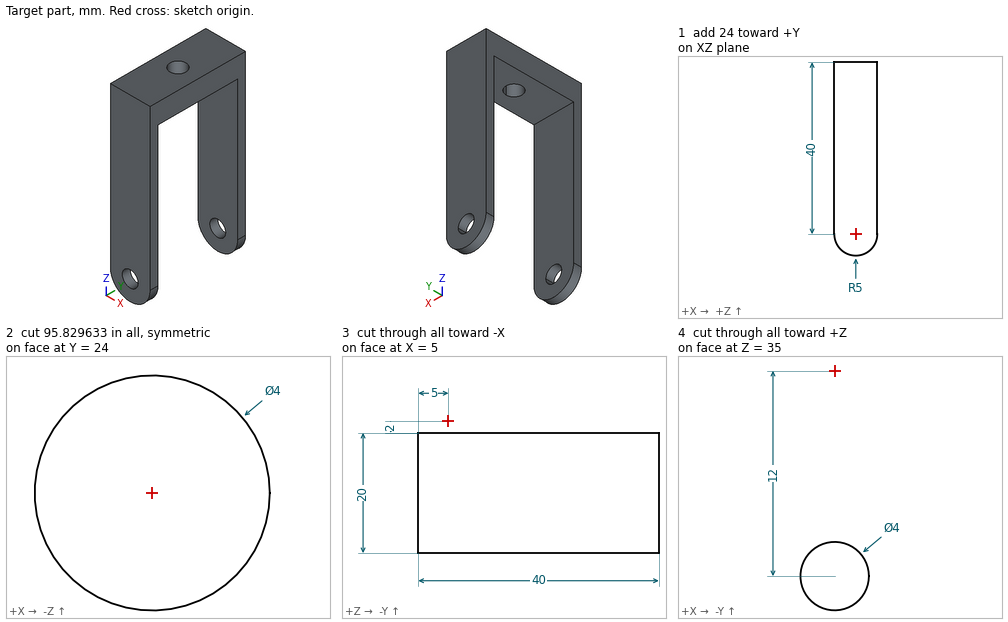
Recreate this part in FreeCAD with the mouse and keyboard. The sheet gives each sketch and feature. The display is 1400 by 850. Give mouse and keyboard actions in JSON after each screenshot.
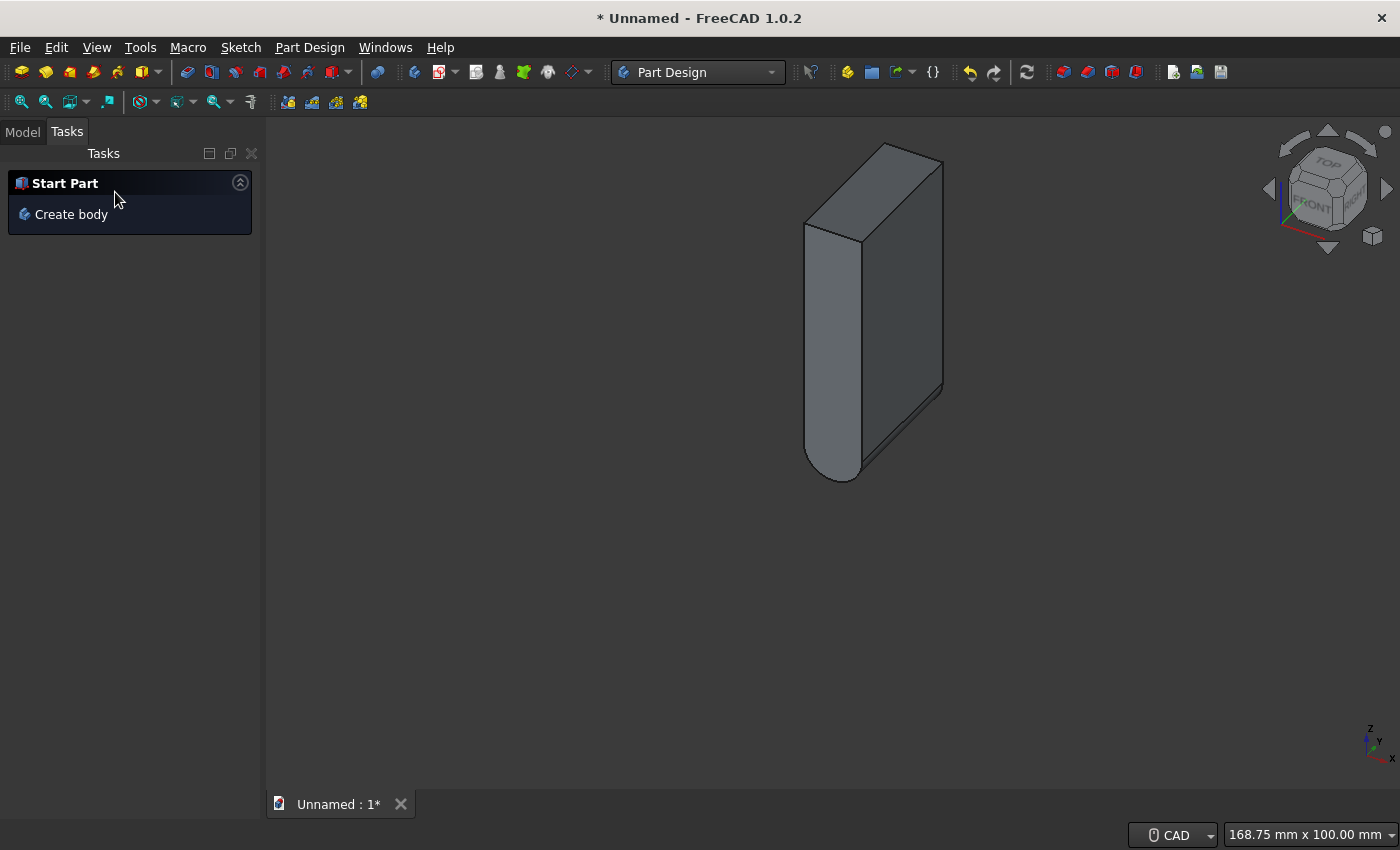
{"action": "key", "text": "4"}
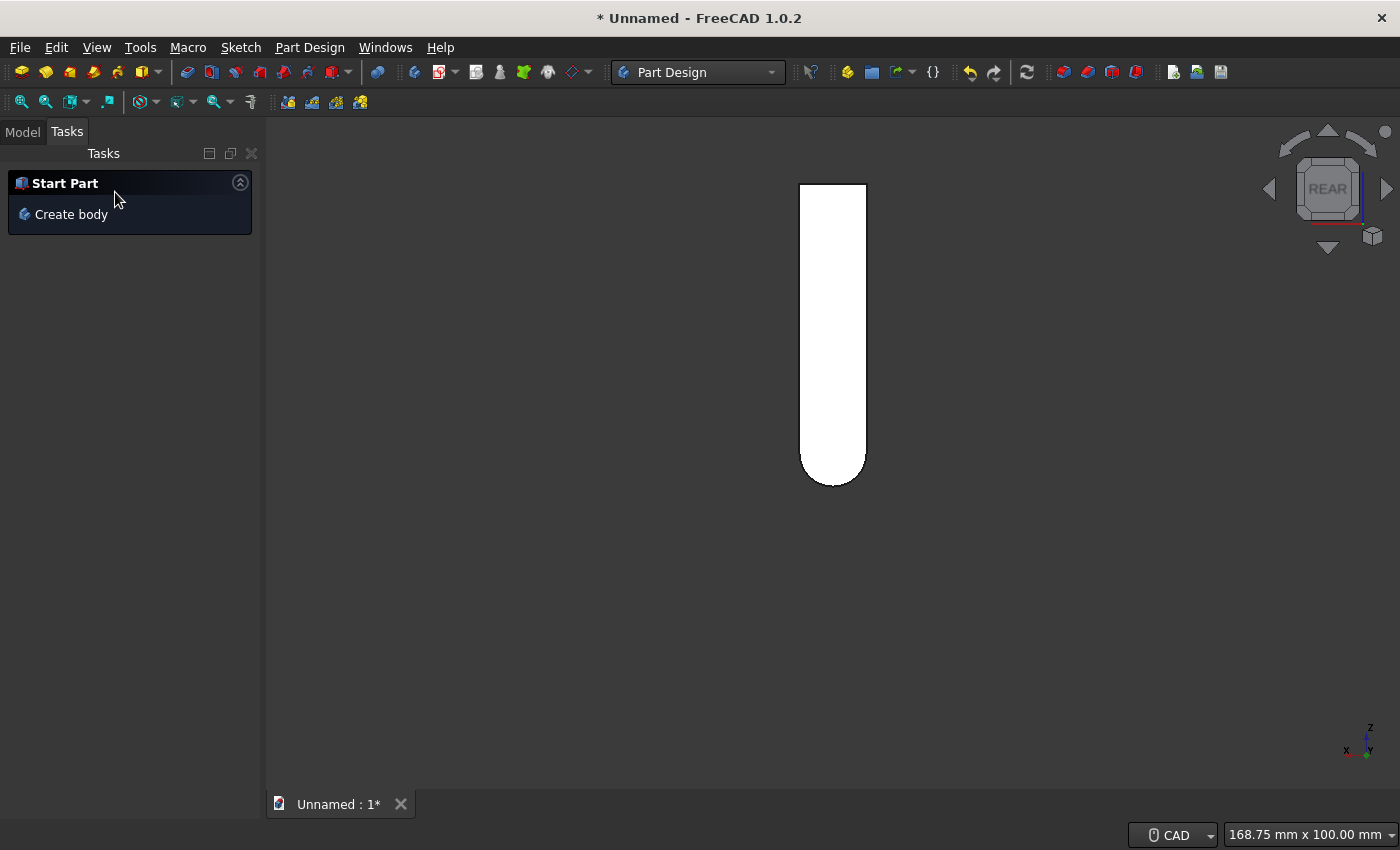
{"action": "left_click", "coordinate": [833, 248]}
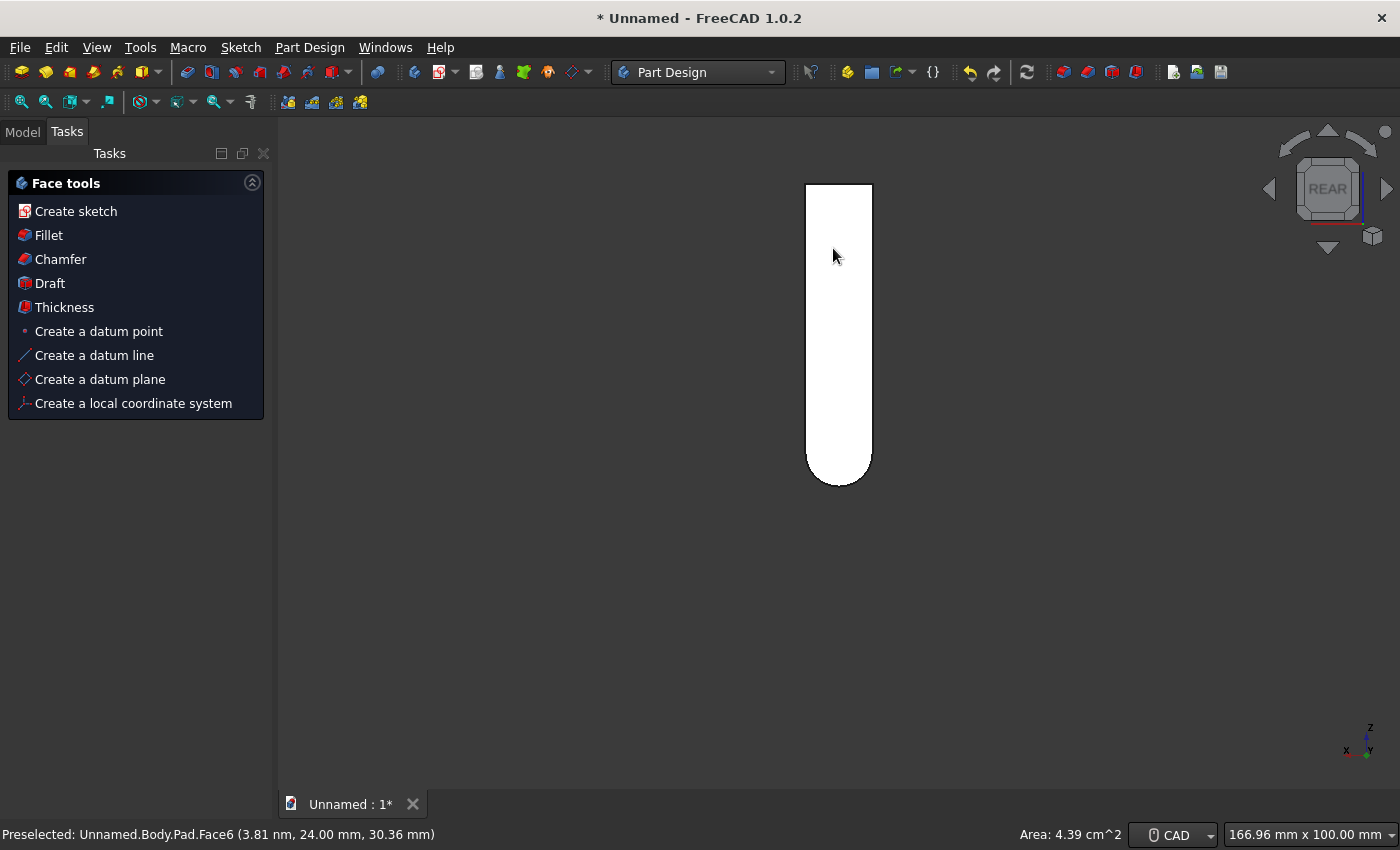
{"action": "left_click", "coordinate": [440, 72]}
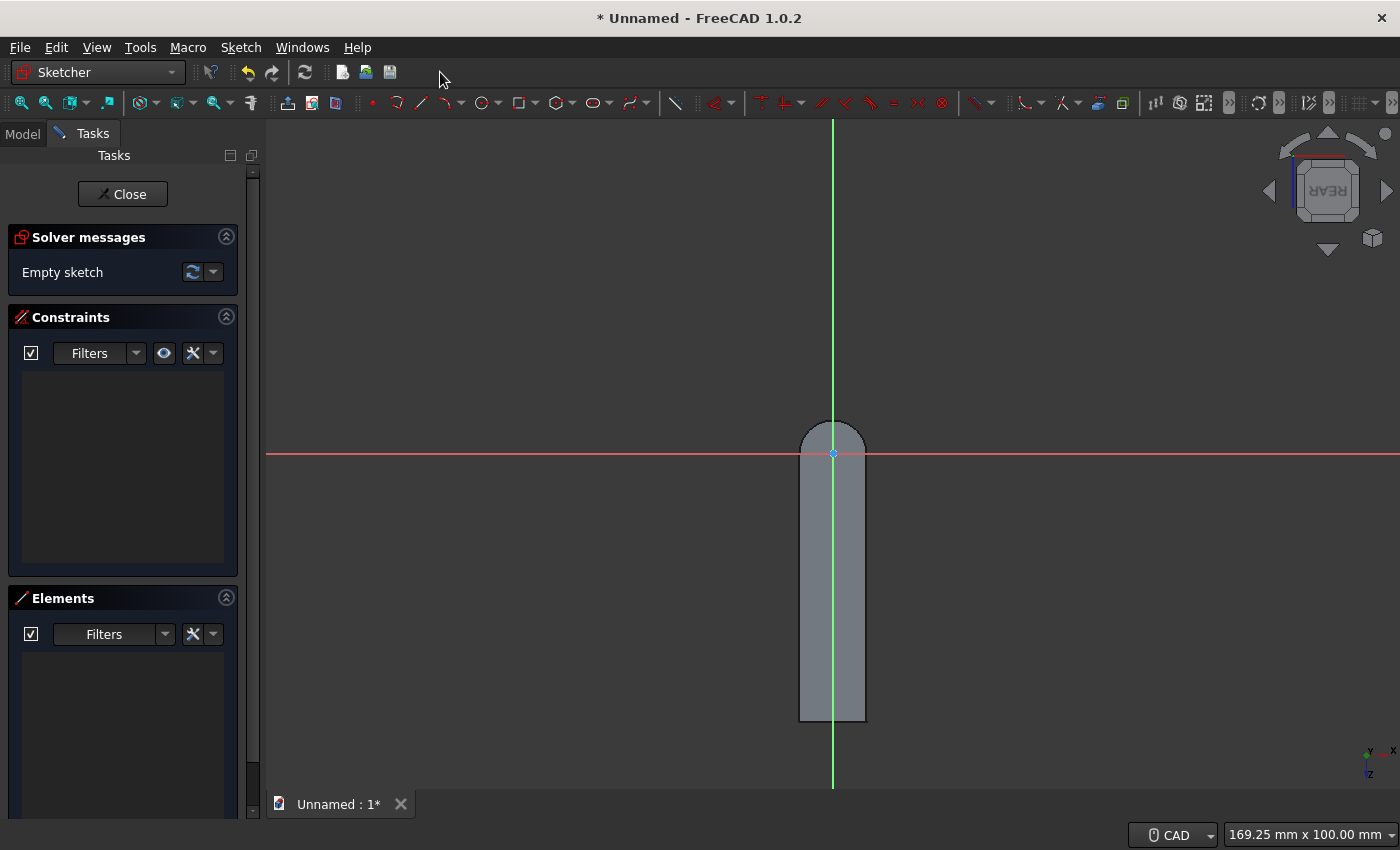
{"action": "scroll", "coordinate": [837, 454], "scroll_direction": "up", "scroll_amount": 14}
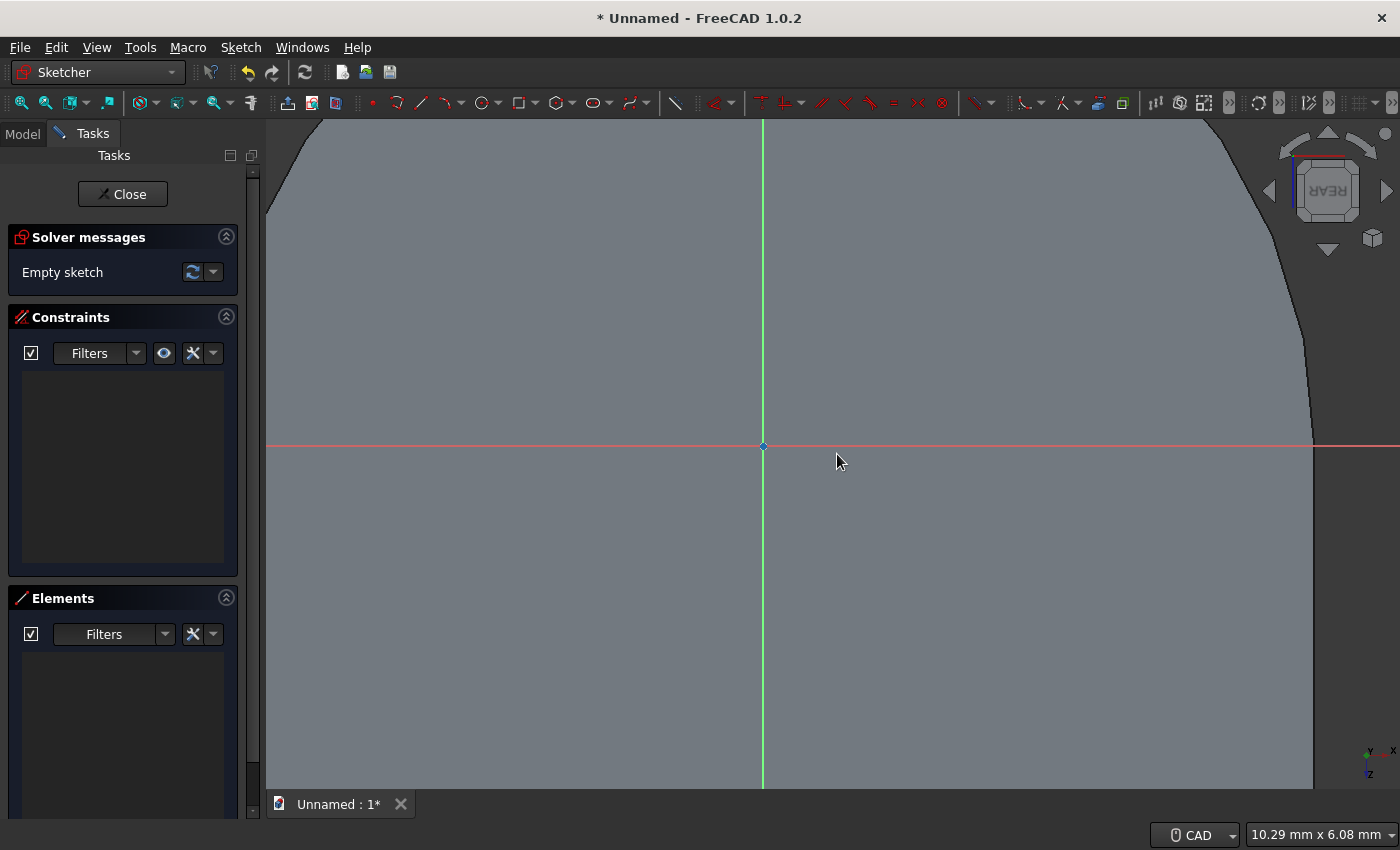
{"action": "key", "text": "g c"}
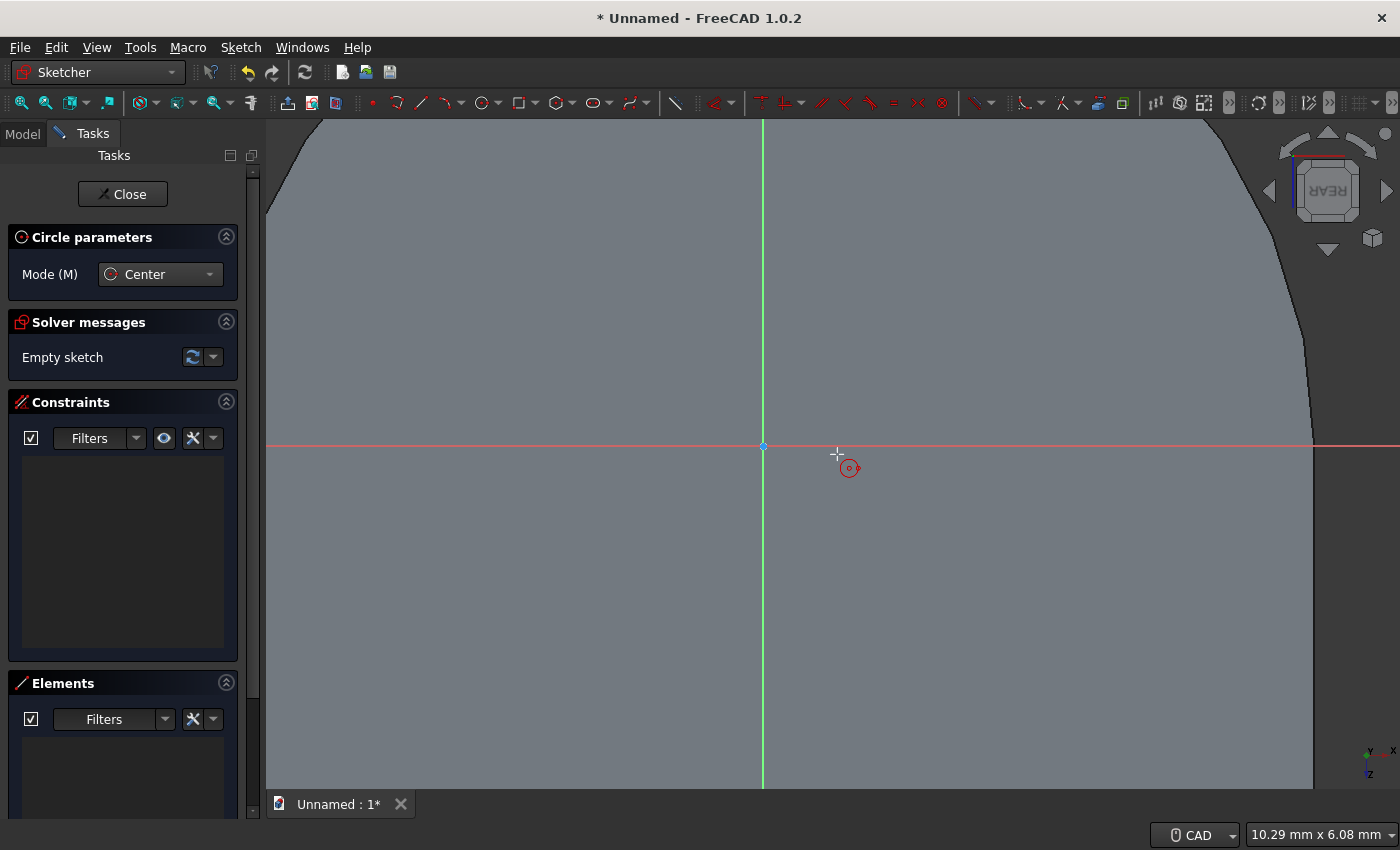
{"action": "left_click", "coordinate": [763, 446]}
{"action": "left_click", "coordinate": [919, 290]}
{"action": "key", "text": "Escape"}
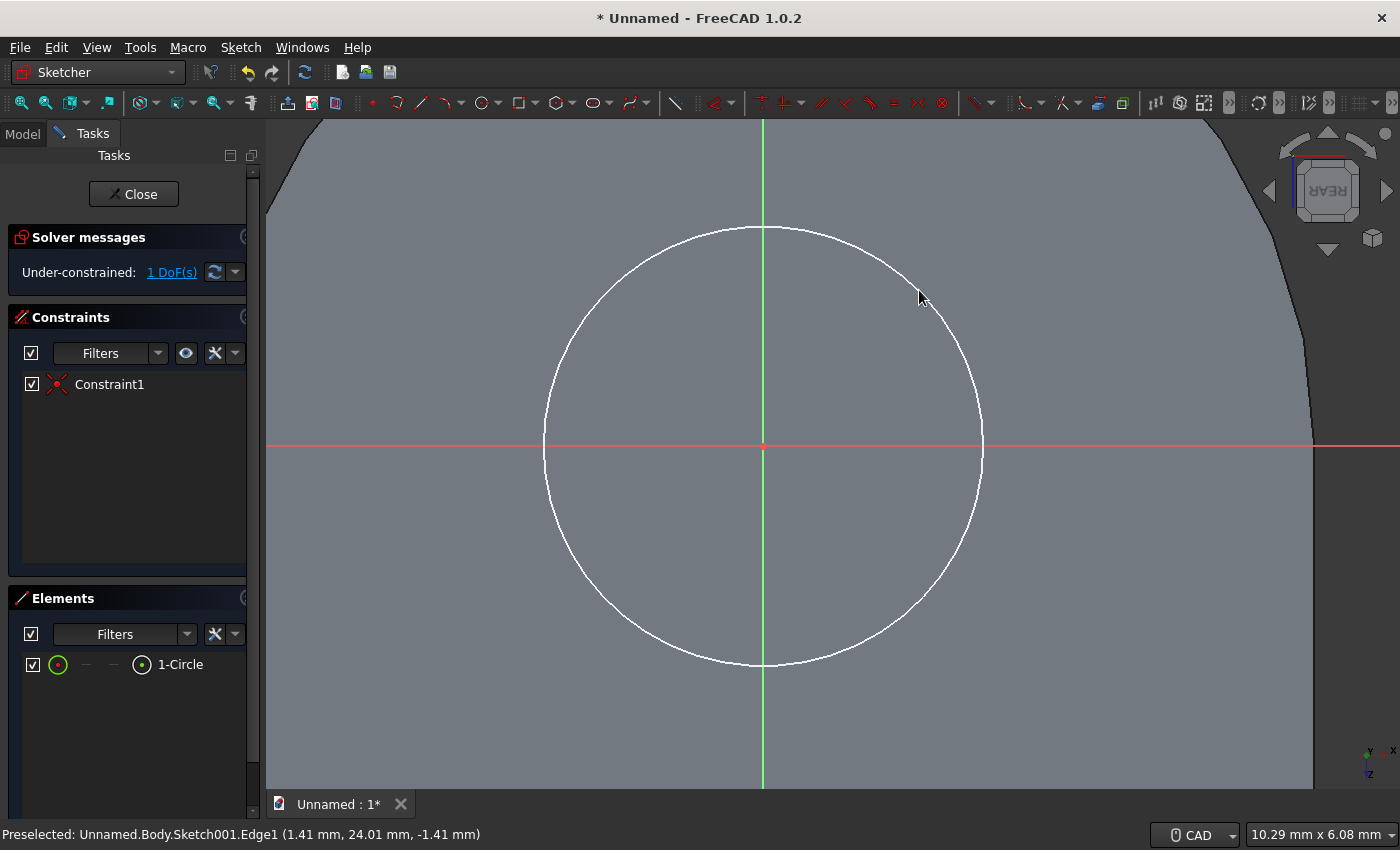
{"action": "left_click", "coordinate": [918, 290]}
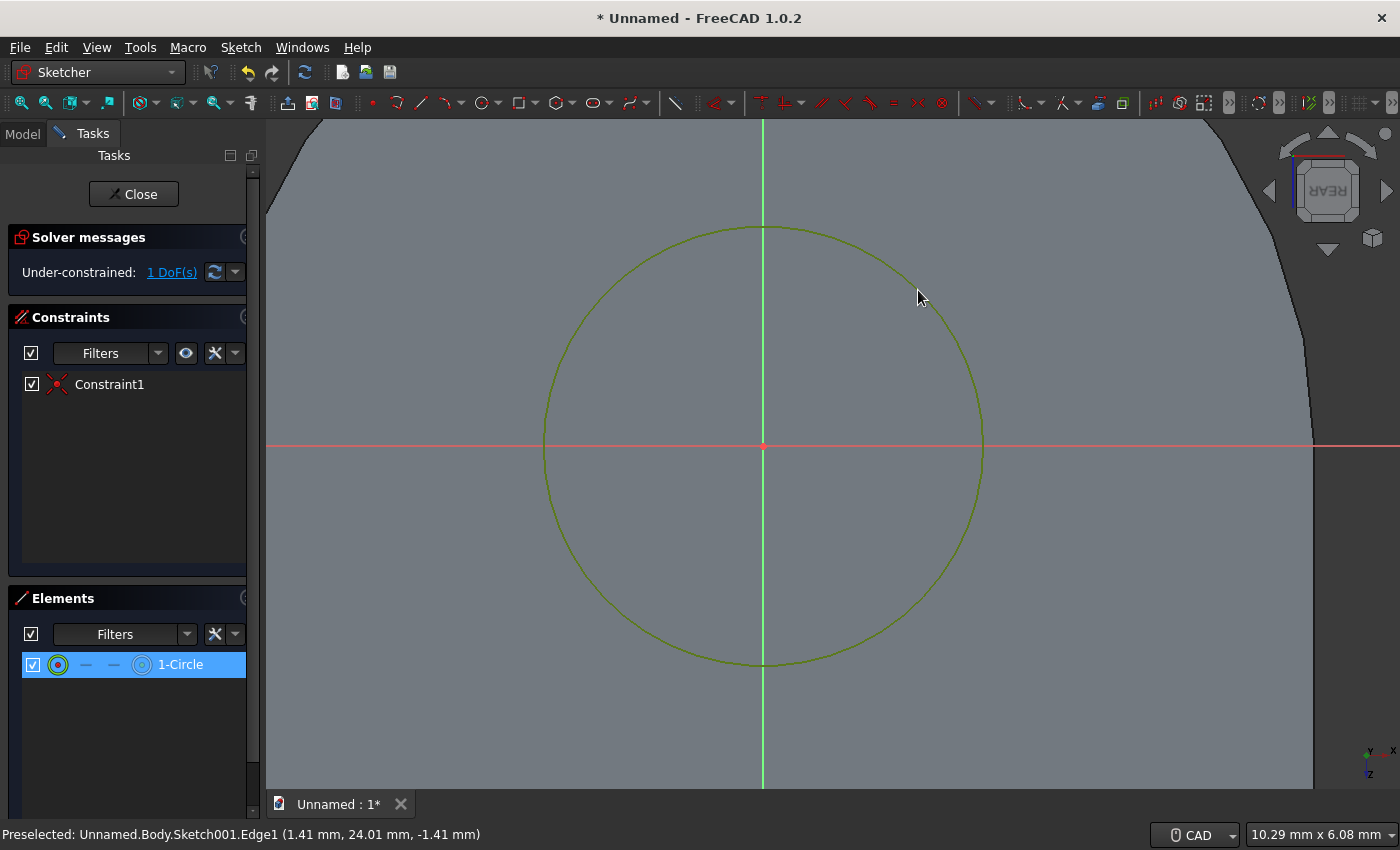
{"action": "left_click", "coordinate": [734, 104]}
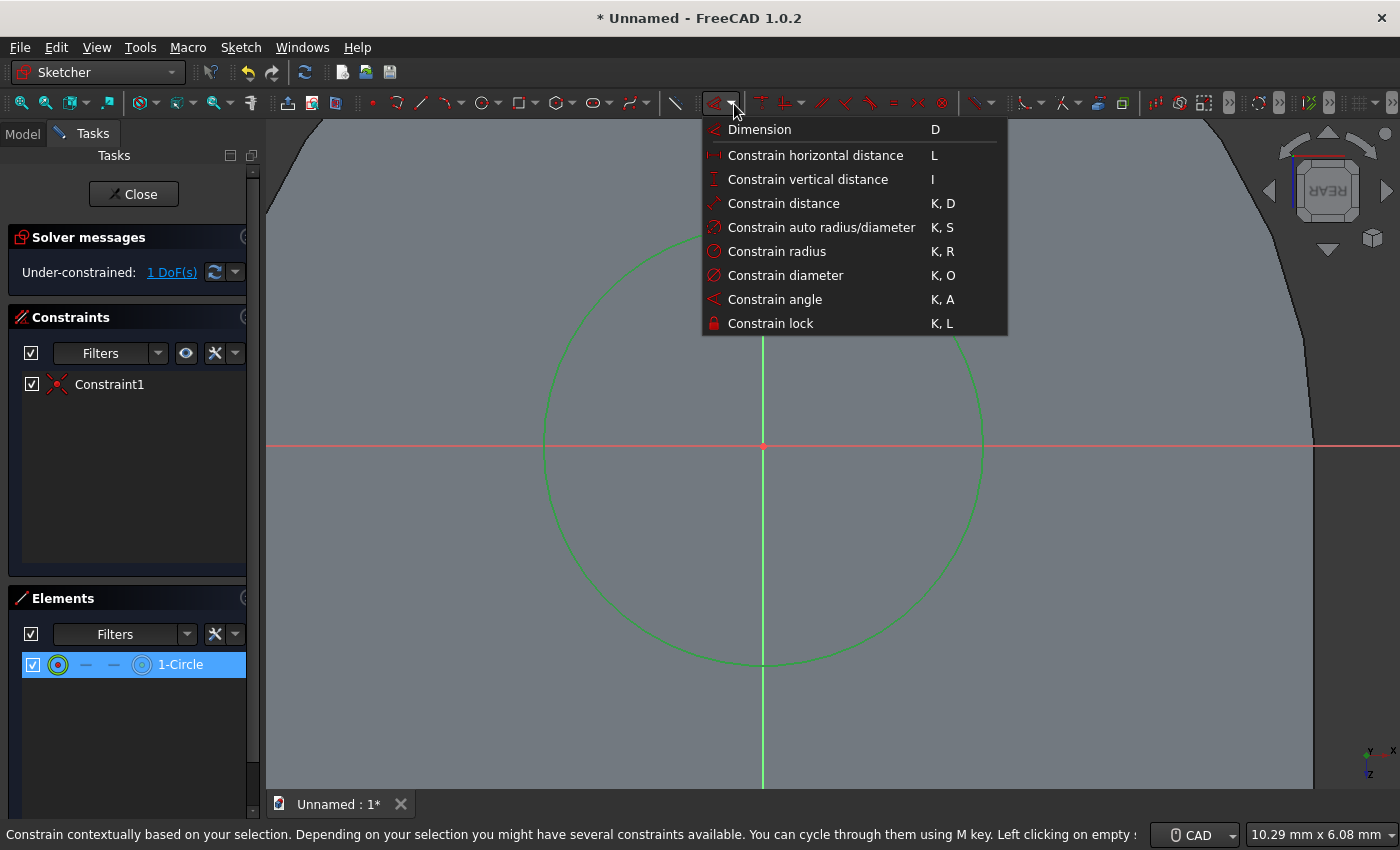
{"action": "left_click", "coordinate": [855, 275]}